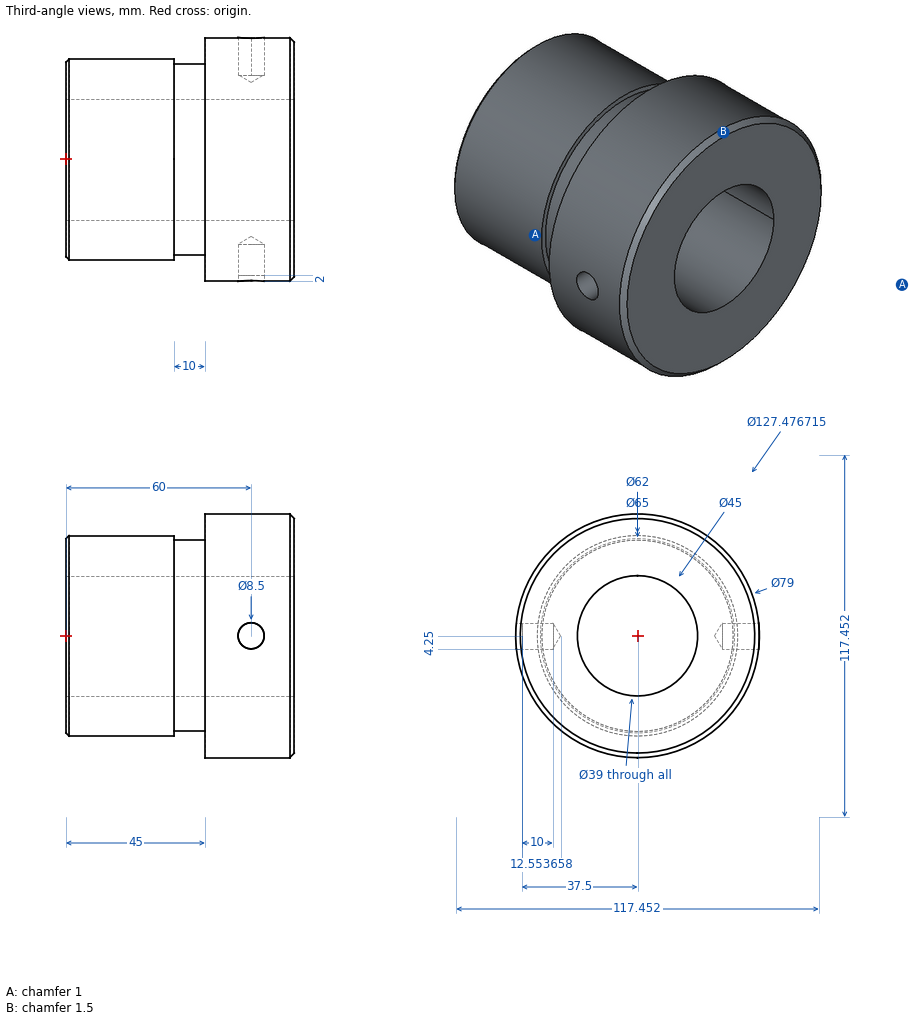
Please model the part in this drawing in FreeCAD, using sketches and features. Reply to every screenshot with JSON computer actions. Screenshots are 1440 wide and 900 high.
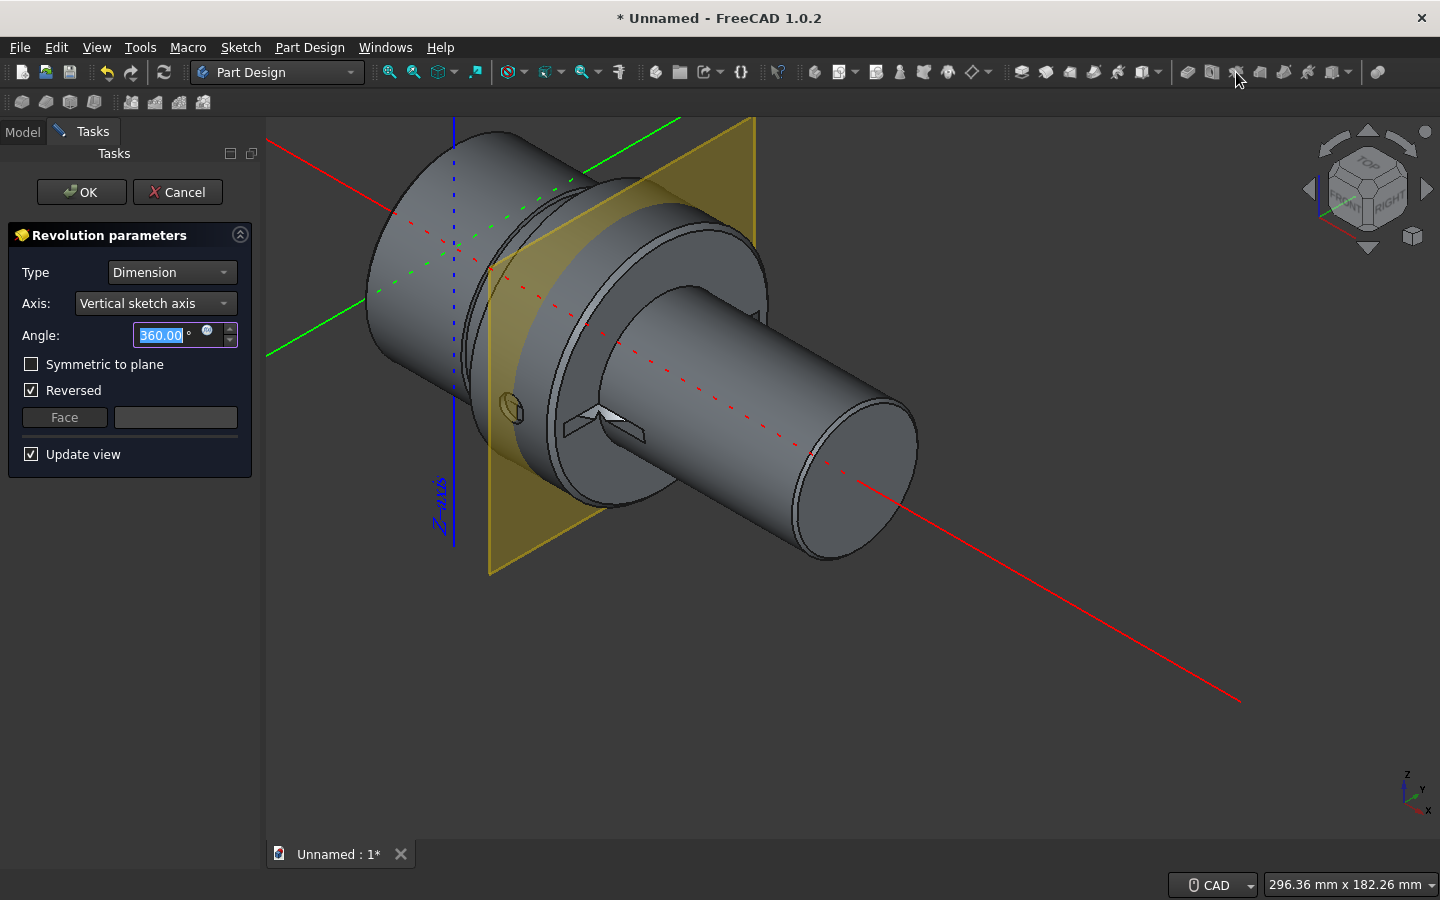
{"action": "left_click", "coordinate": [156, 304]}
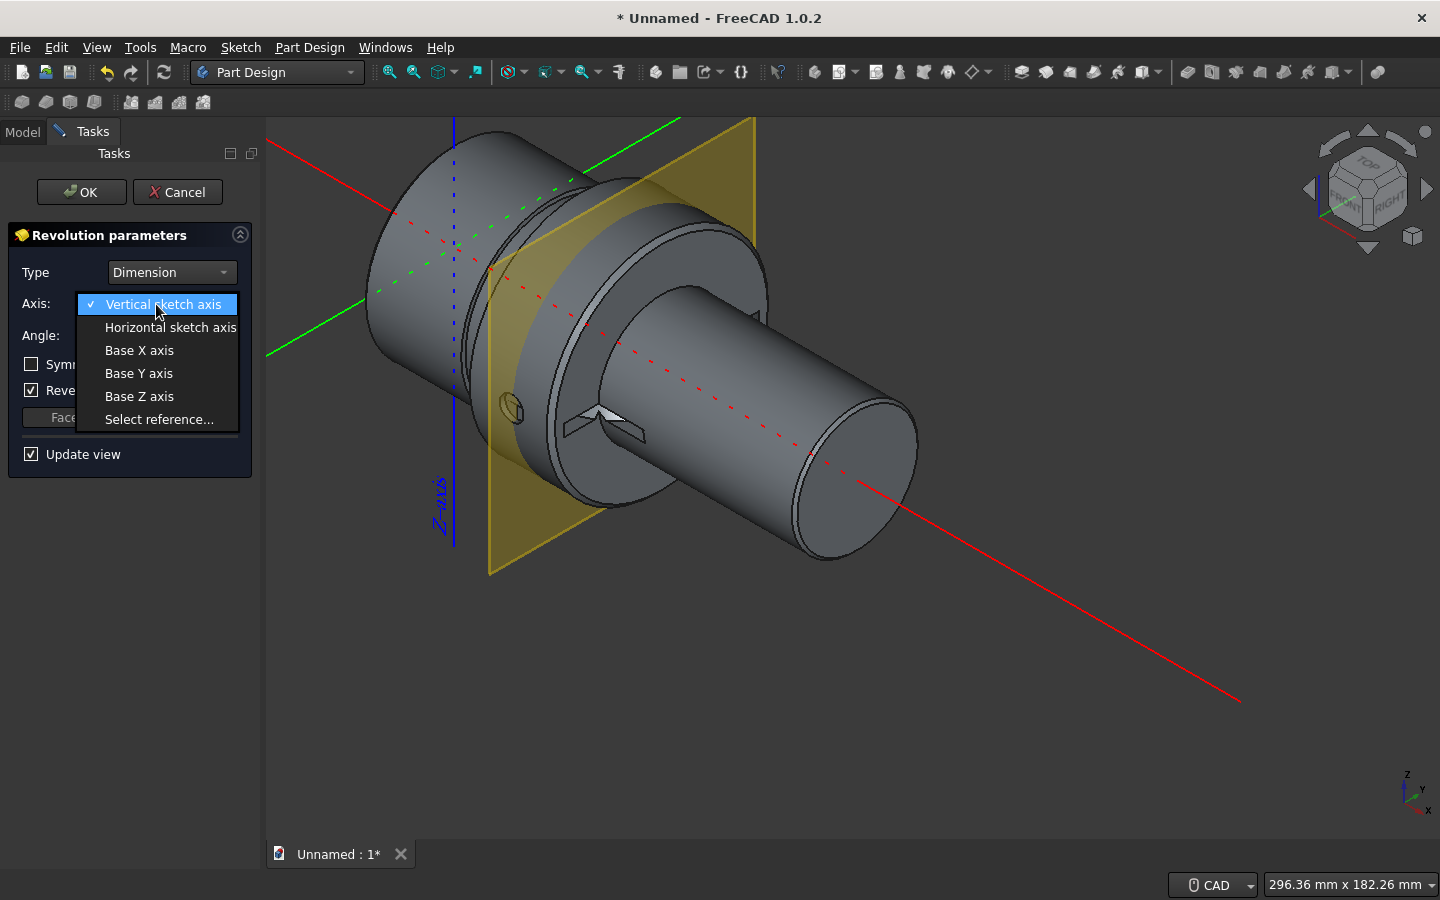
{"action": "left_click", "coordinate": [156, 328]}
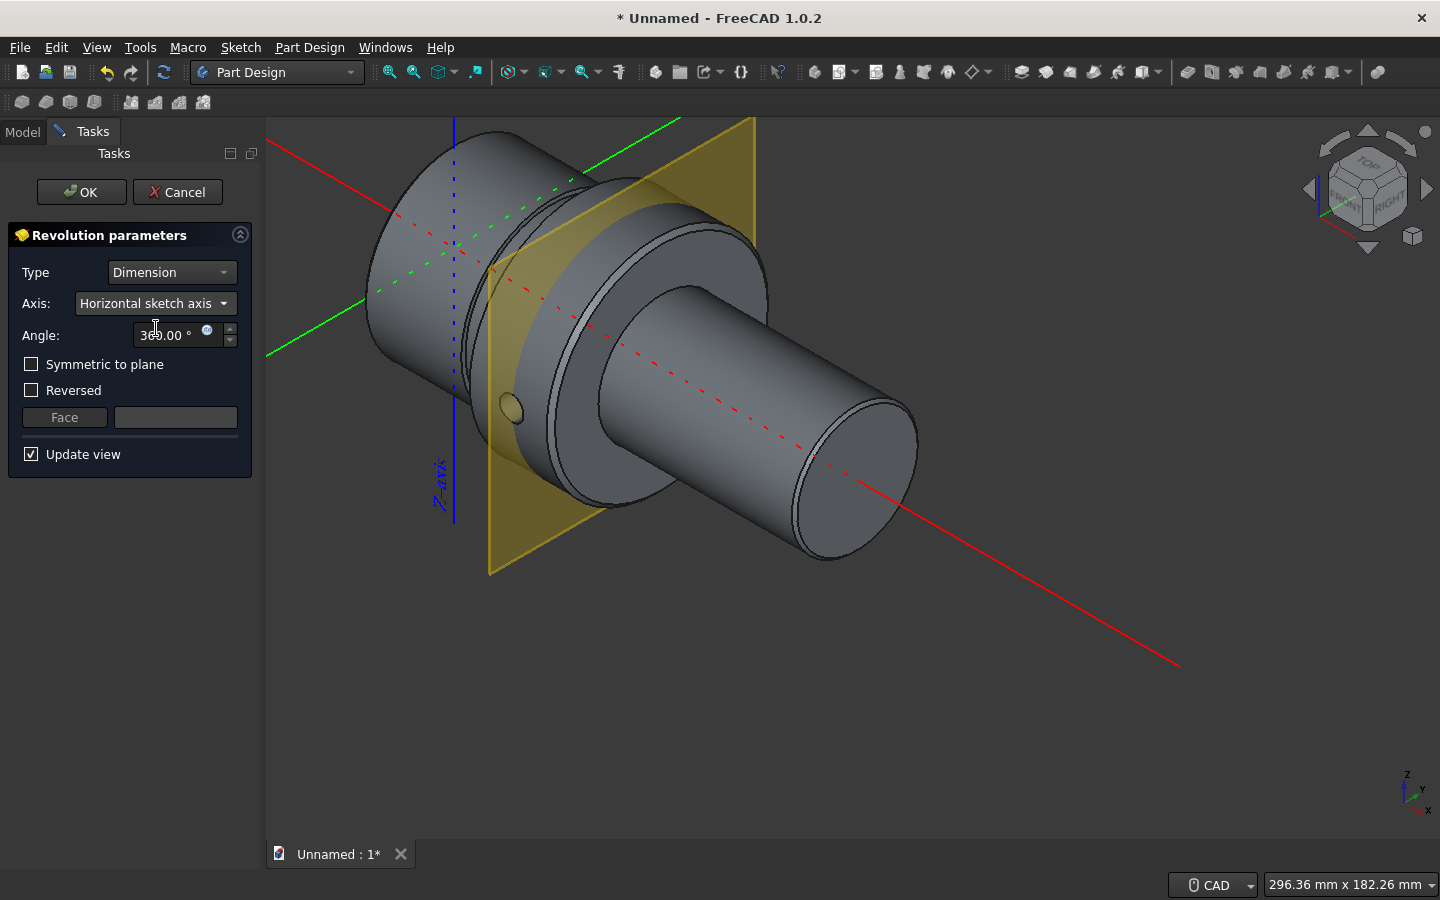
{"action": "left_click", "coordinate": [82, 192]}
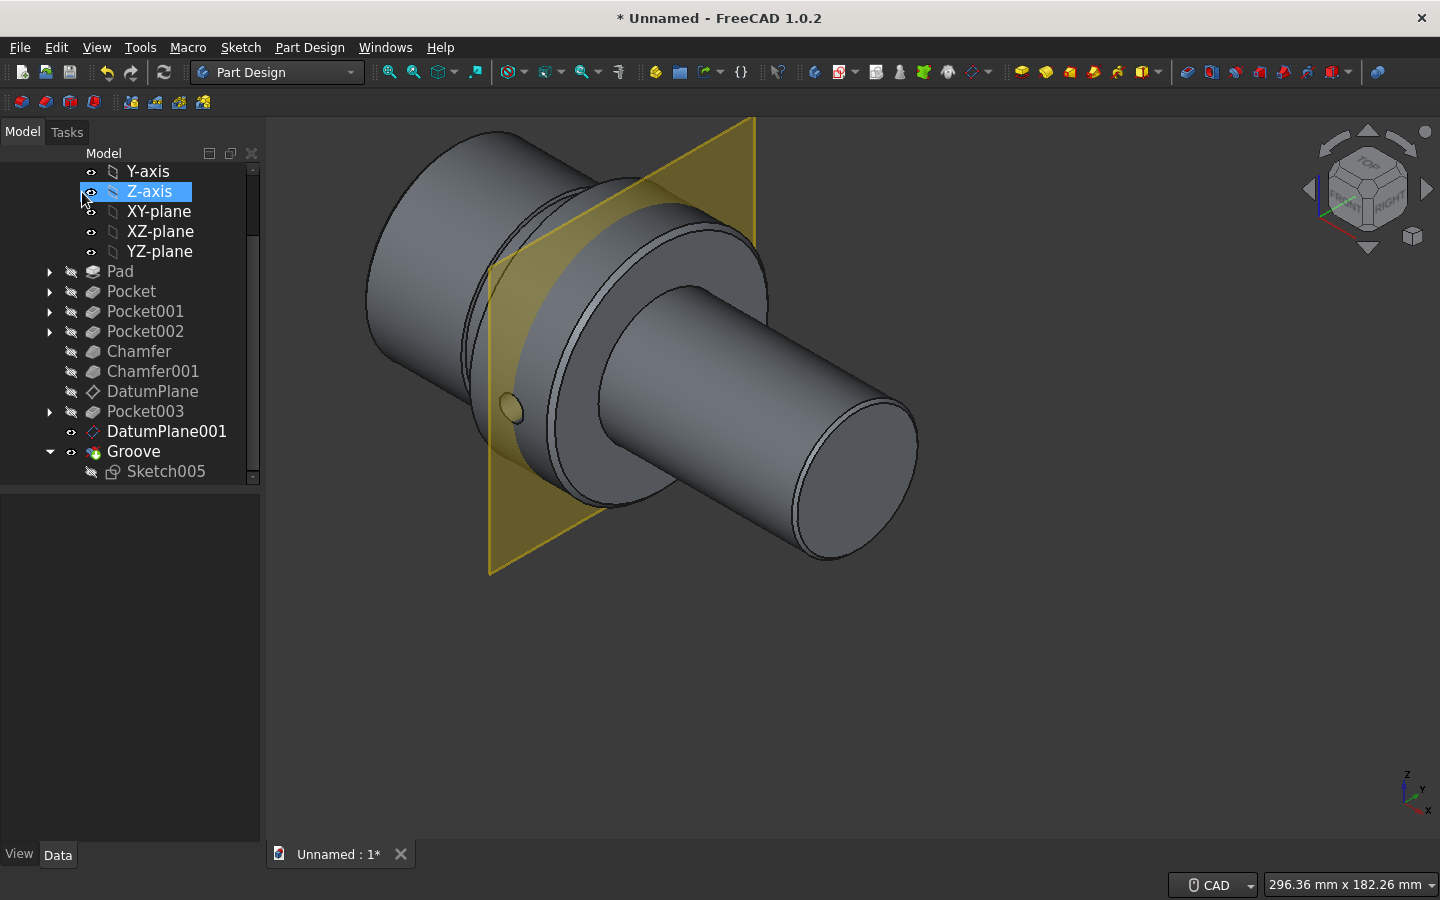
{"action": "left_click", "coordinate": [116, 432]}
{"action": "key", "text": "space"}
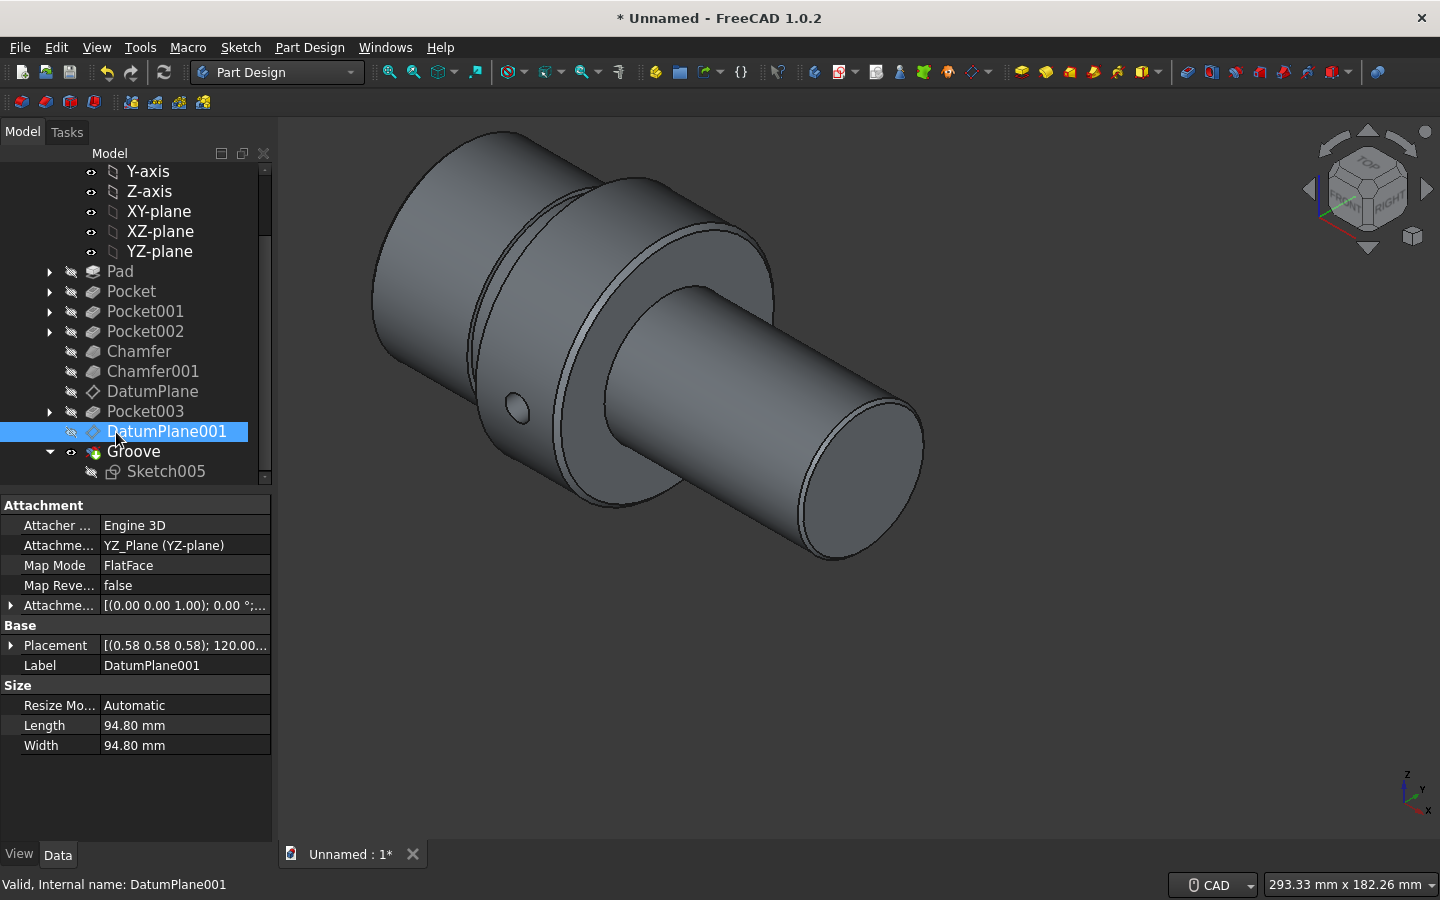
{"action": "key", "text": "v f"}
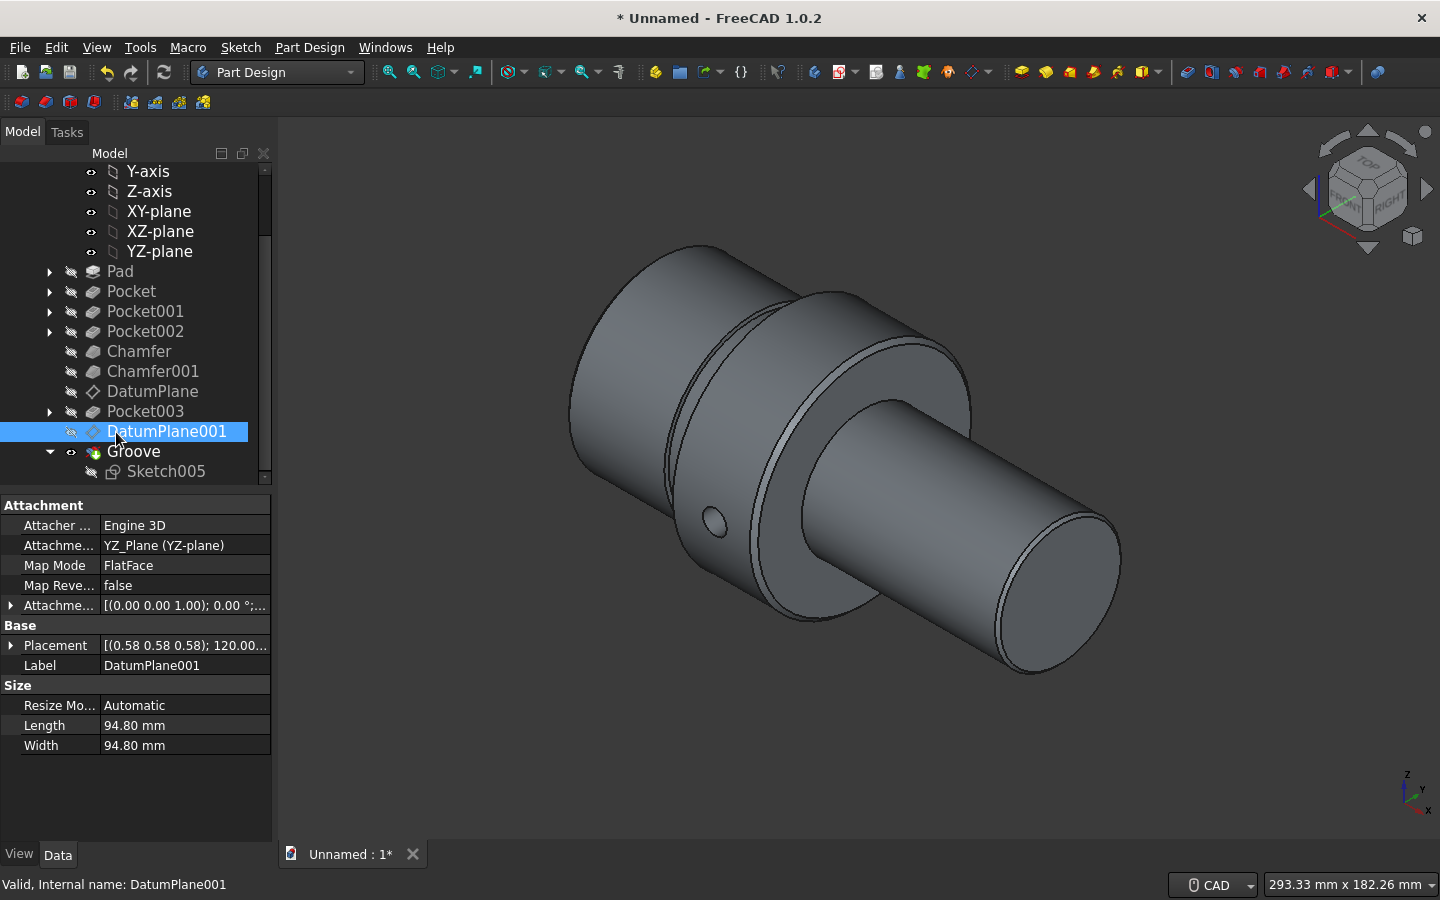
{"action": "left_click", "coordinate": [116, 412]}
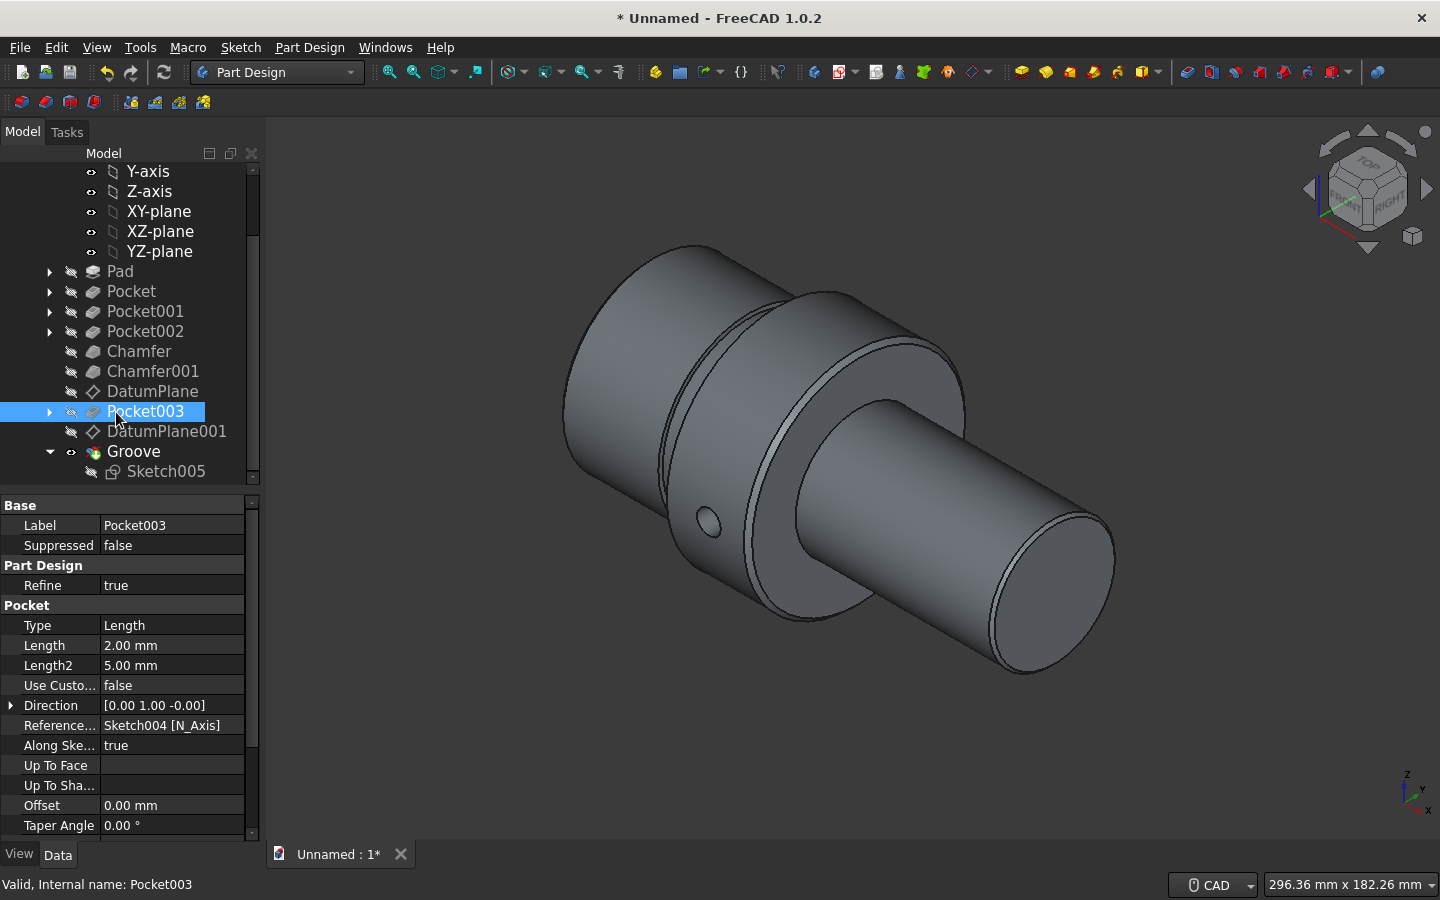
{"action": "left_click", "coordinate": [116, 452], "text": "ctrl"}